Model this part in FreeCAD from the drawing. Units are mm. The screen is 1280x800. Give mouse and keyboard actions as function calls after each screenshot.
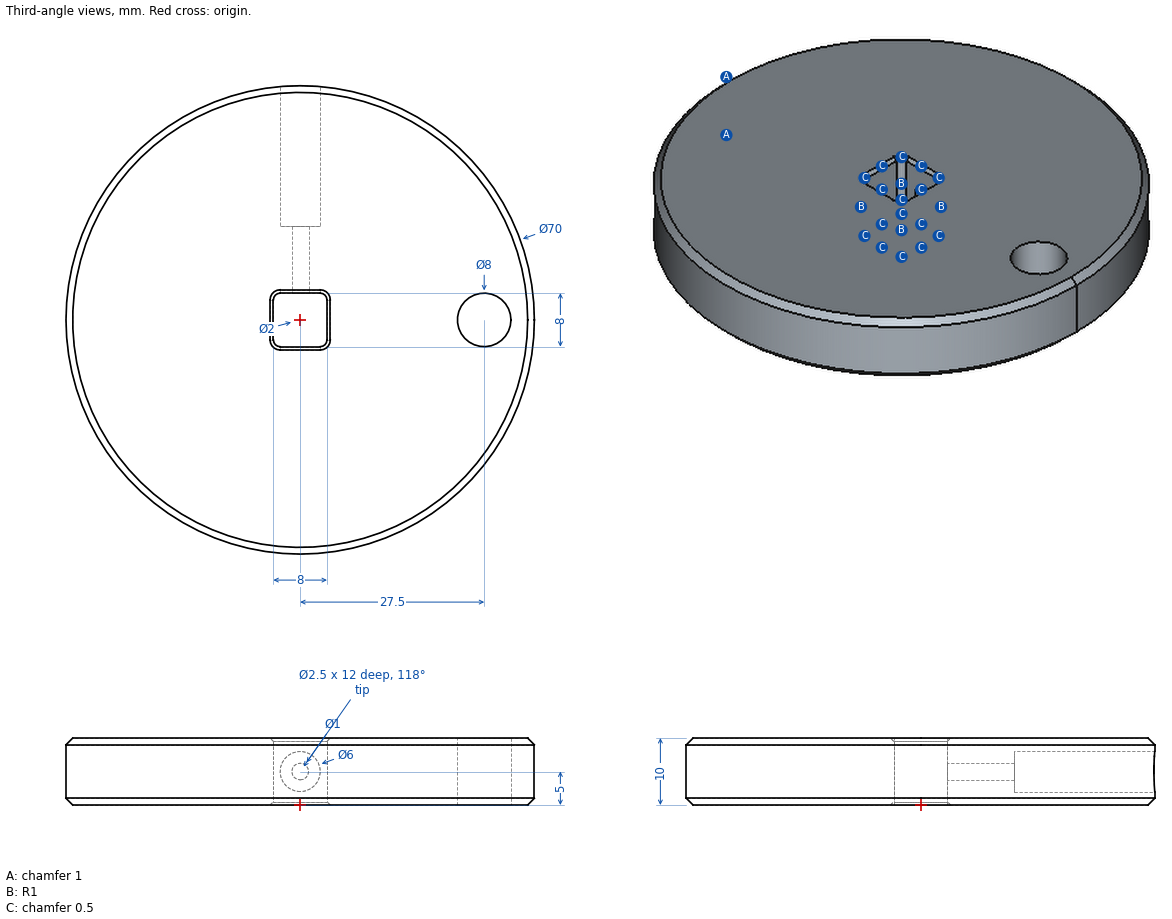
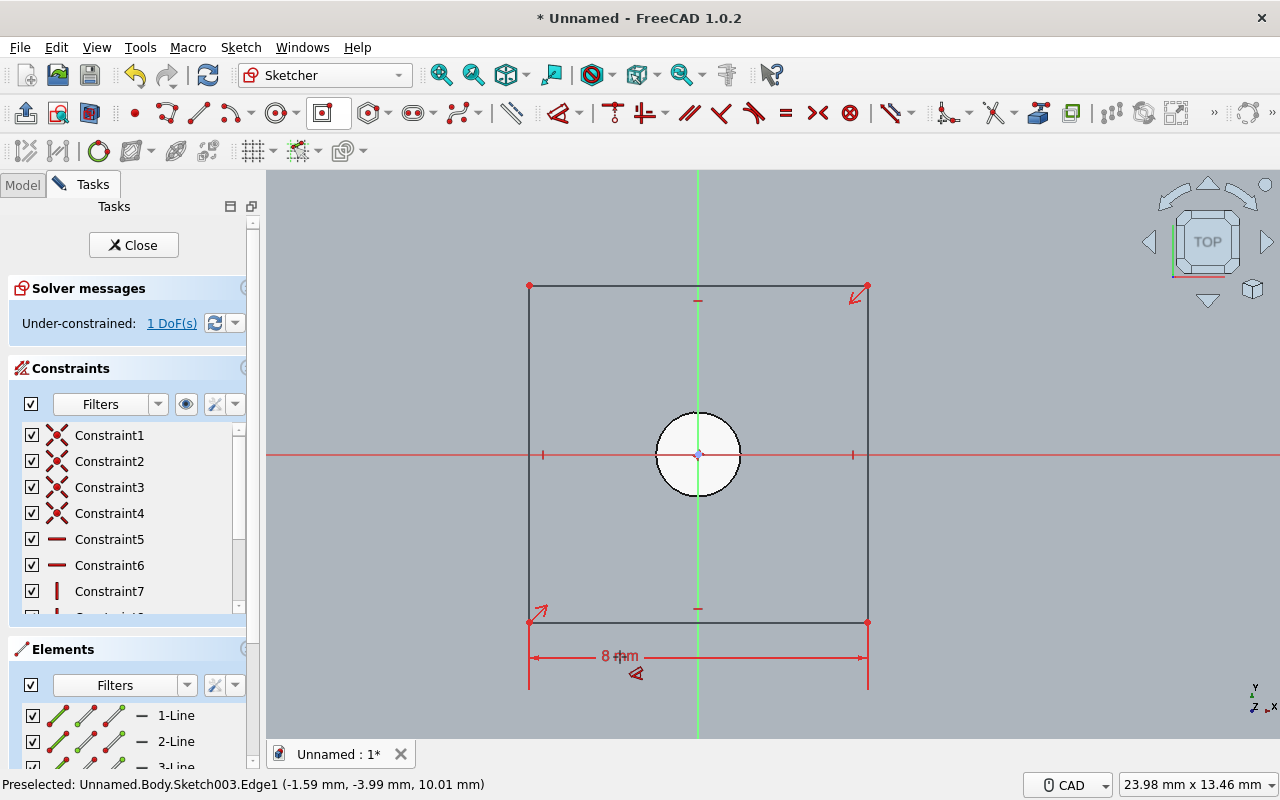
click(868, 522)
click(902, 377)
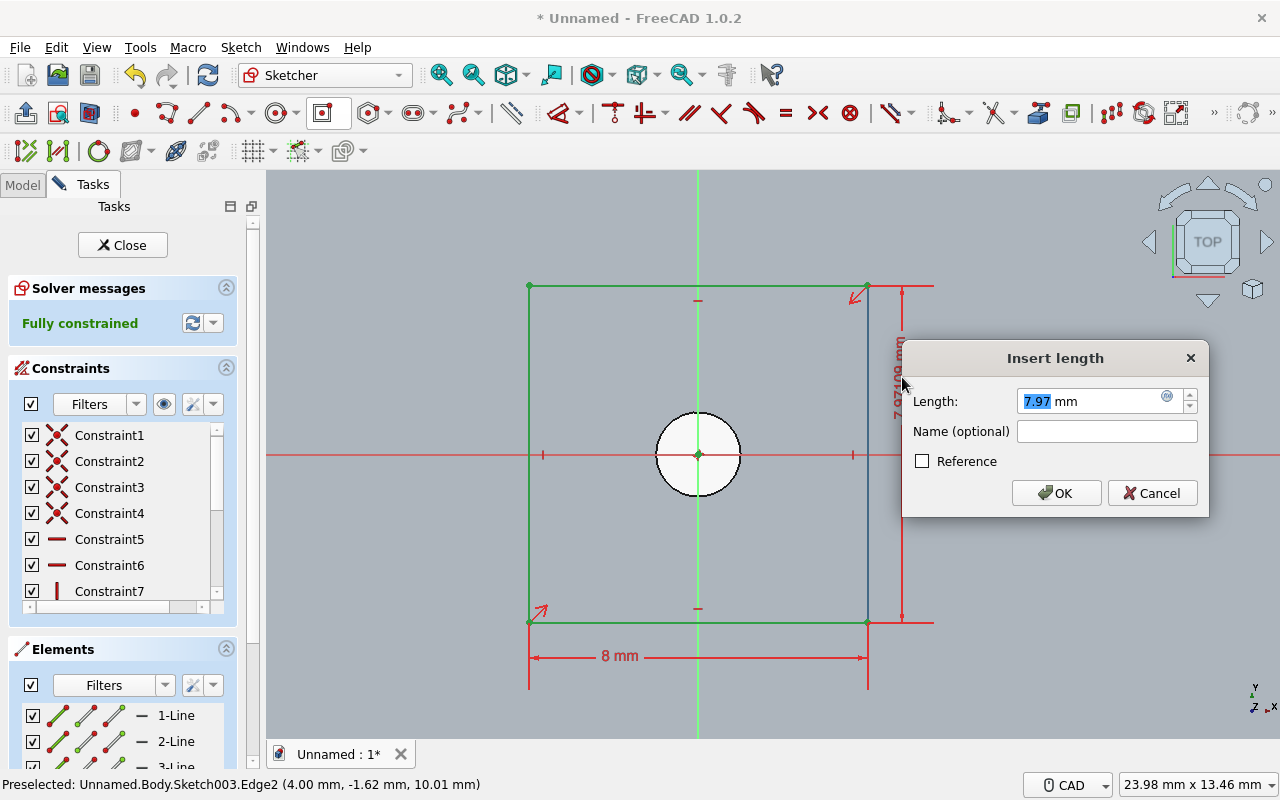
text(8)
key(Return)
key(Escape)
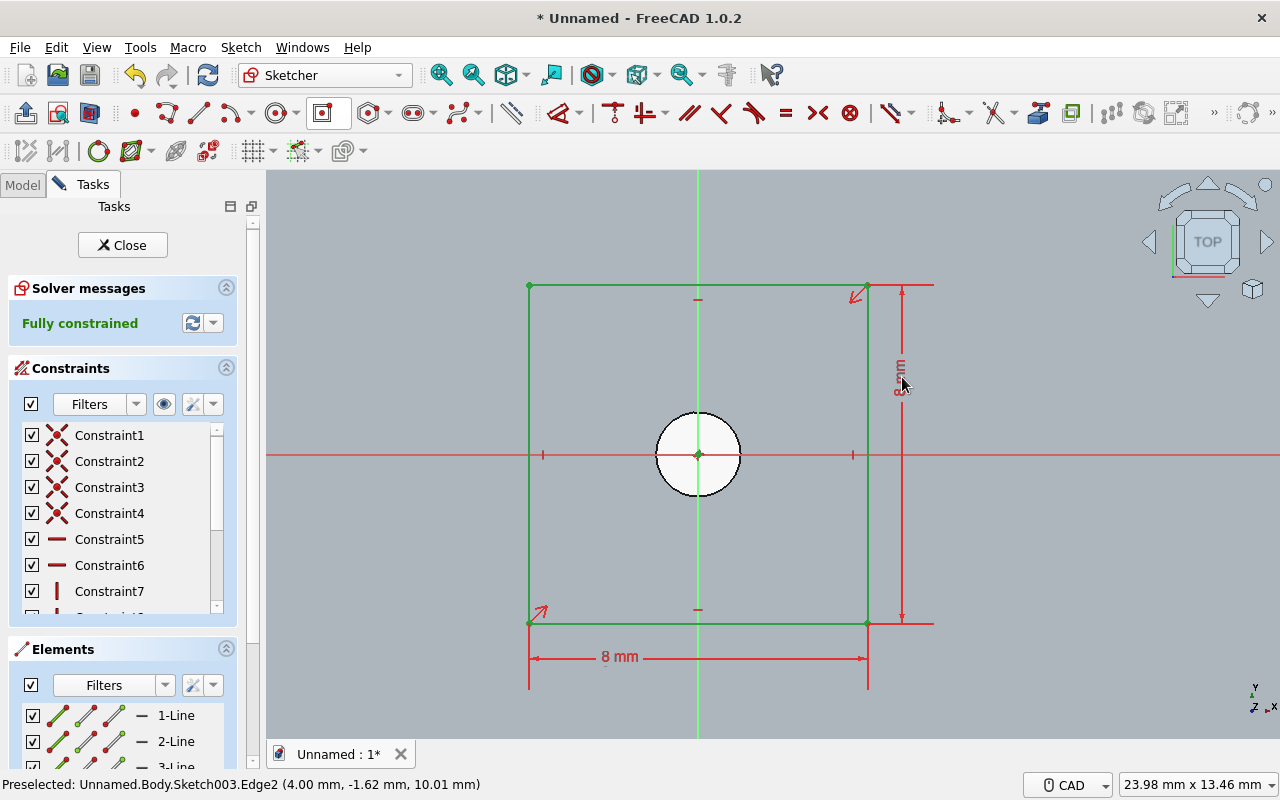
click(123, 245)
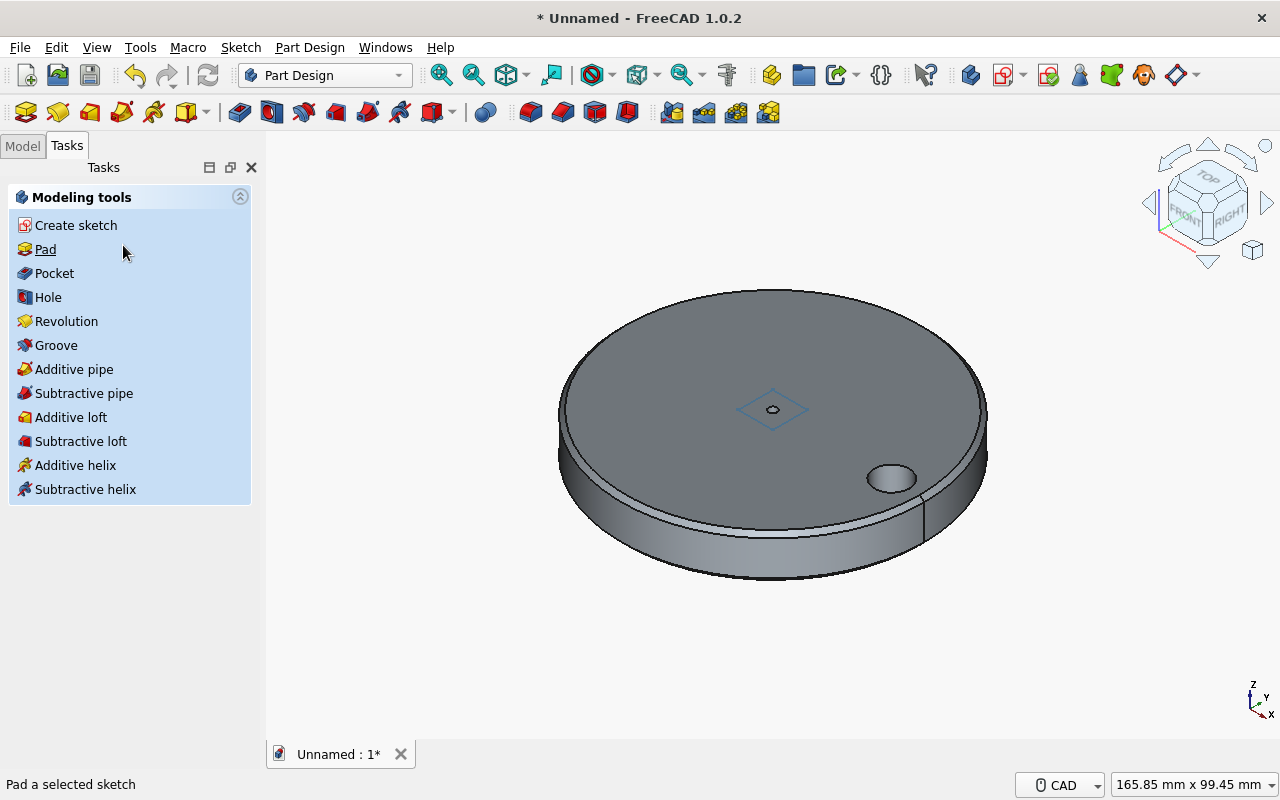
click(240, 112)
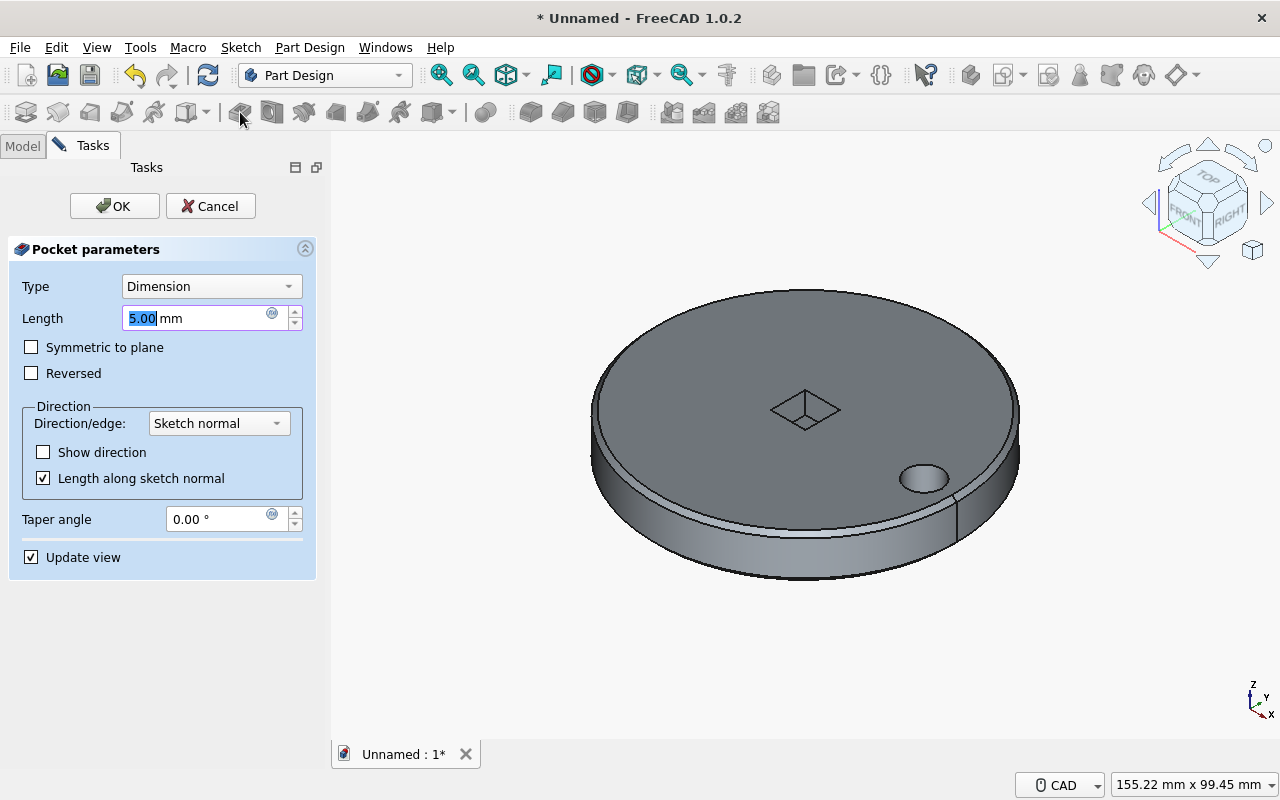
click(212, 286)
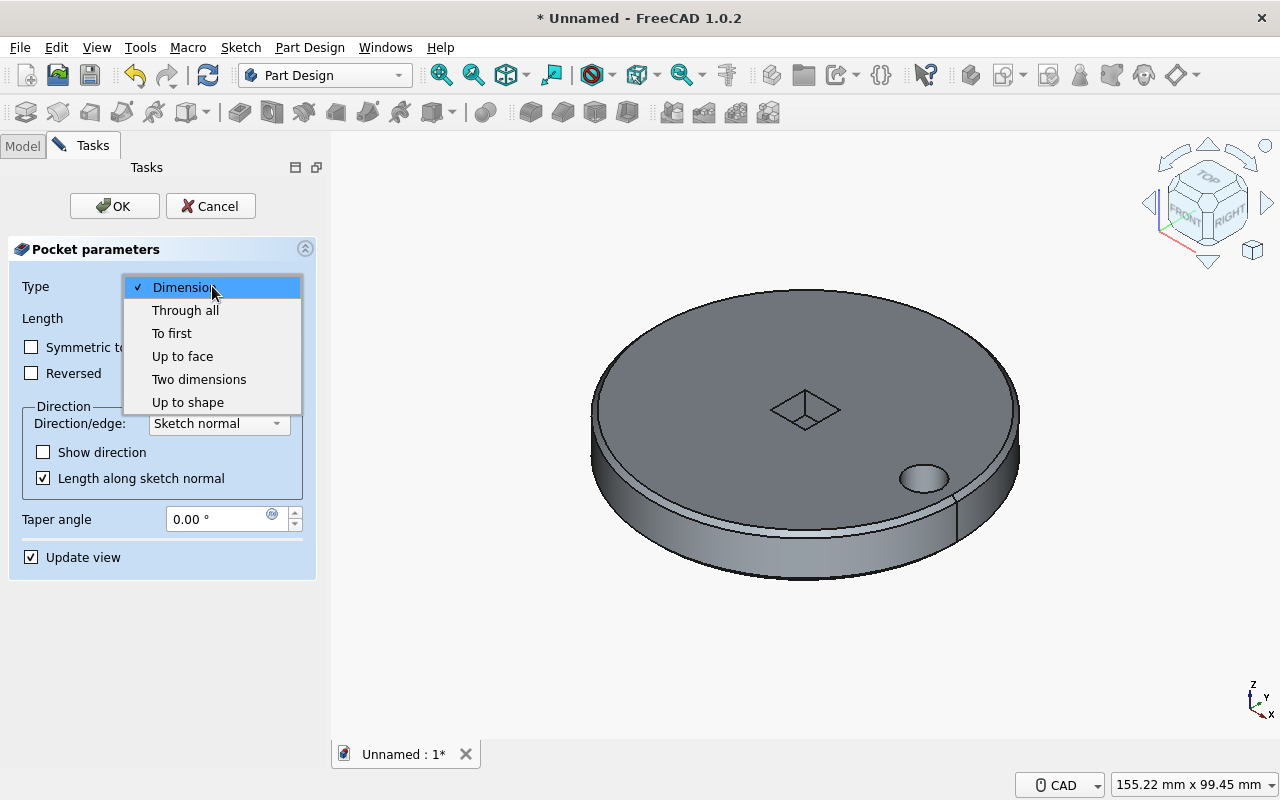
click(212, 310)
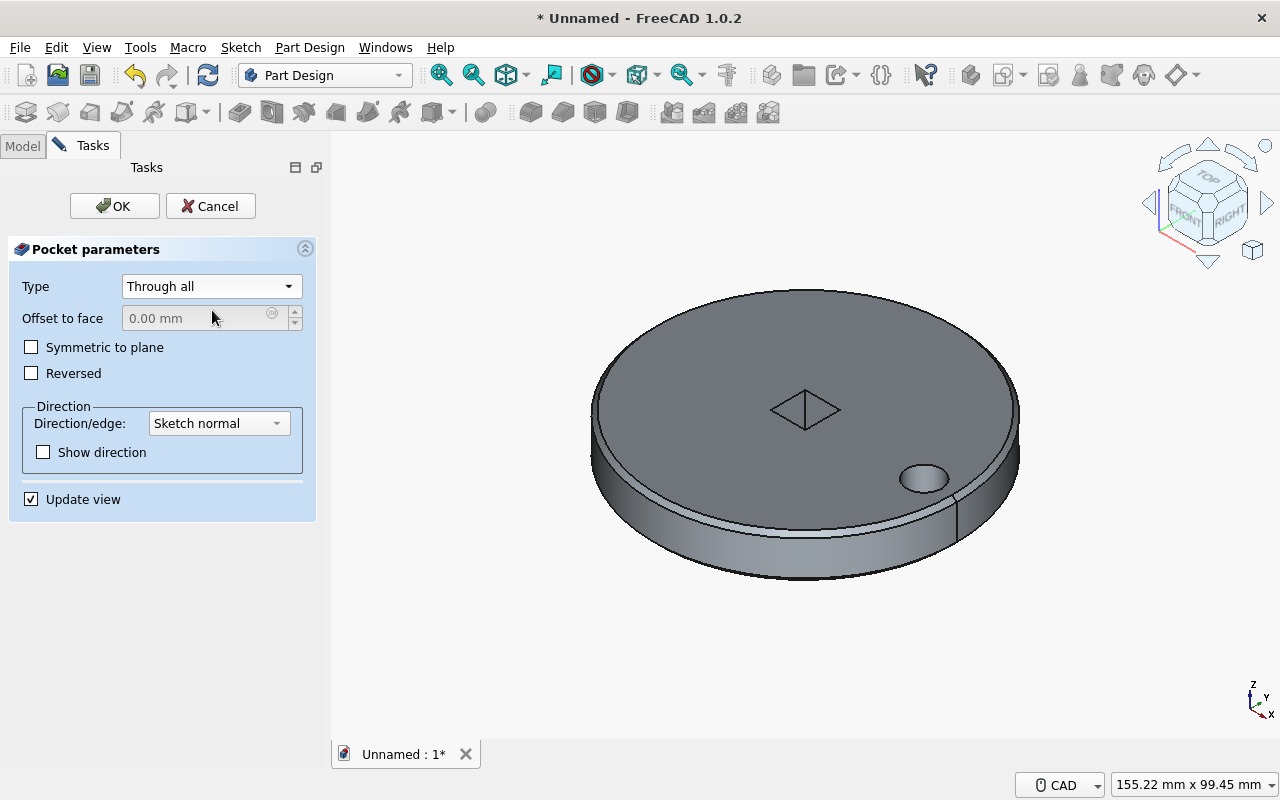
click(115, 206)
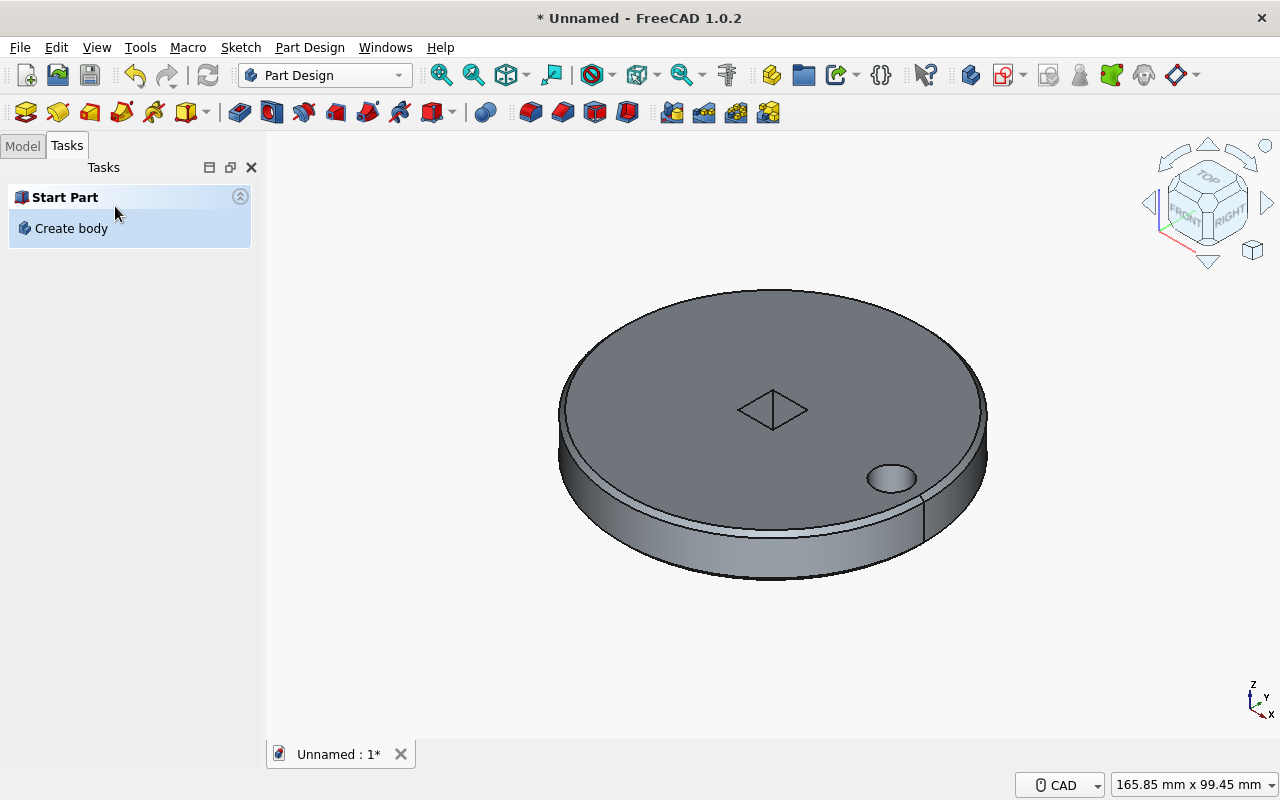
key(2)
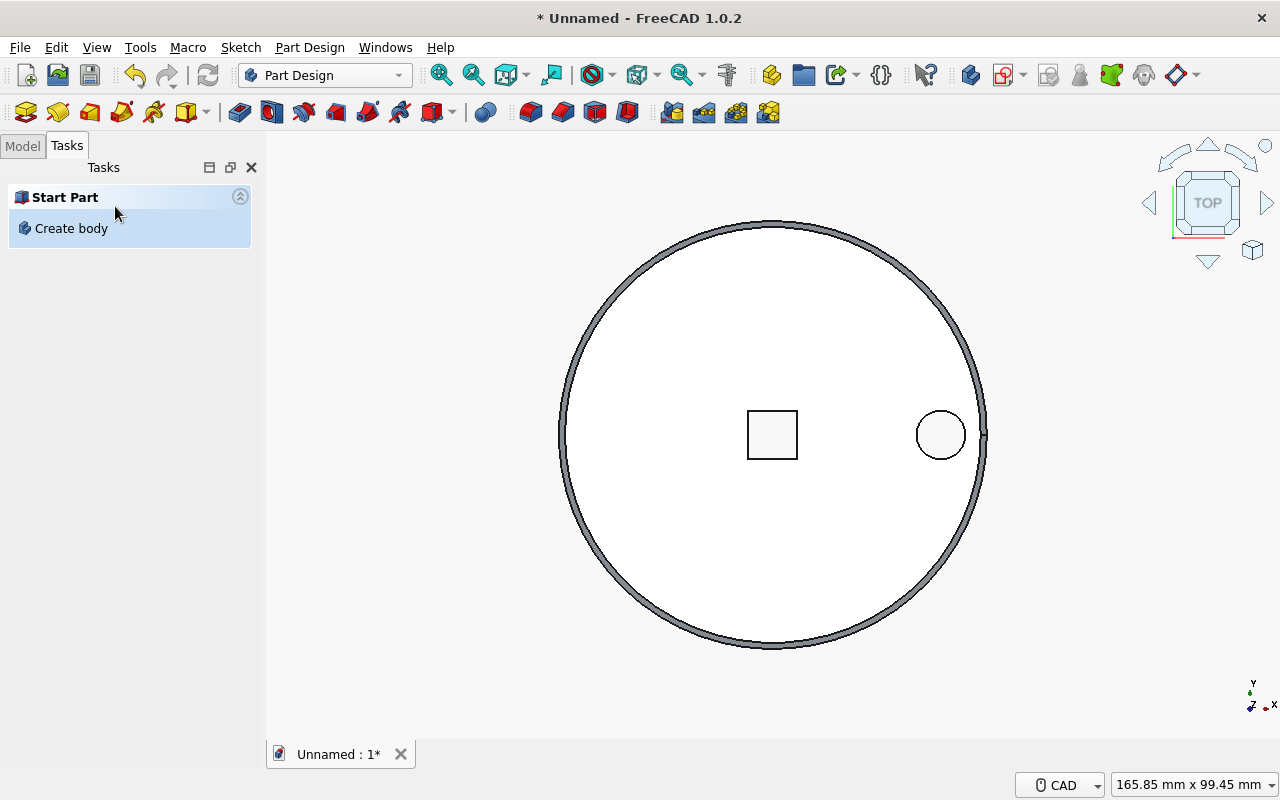
key(0)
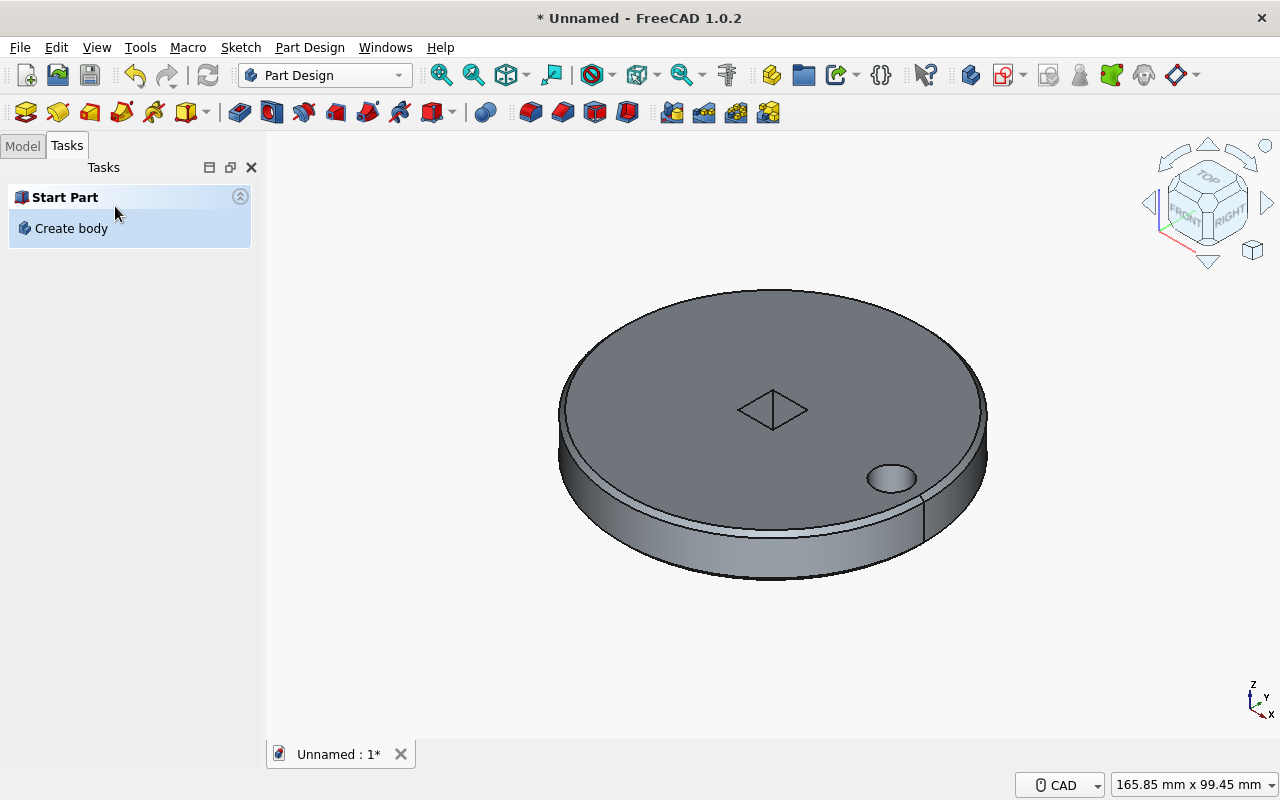
key(1)